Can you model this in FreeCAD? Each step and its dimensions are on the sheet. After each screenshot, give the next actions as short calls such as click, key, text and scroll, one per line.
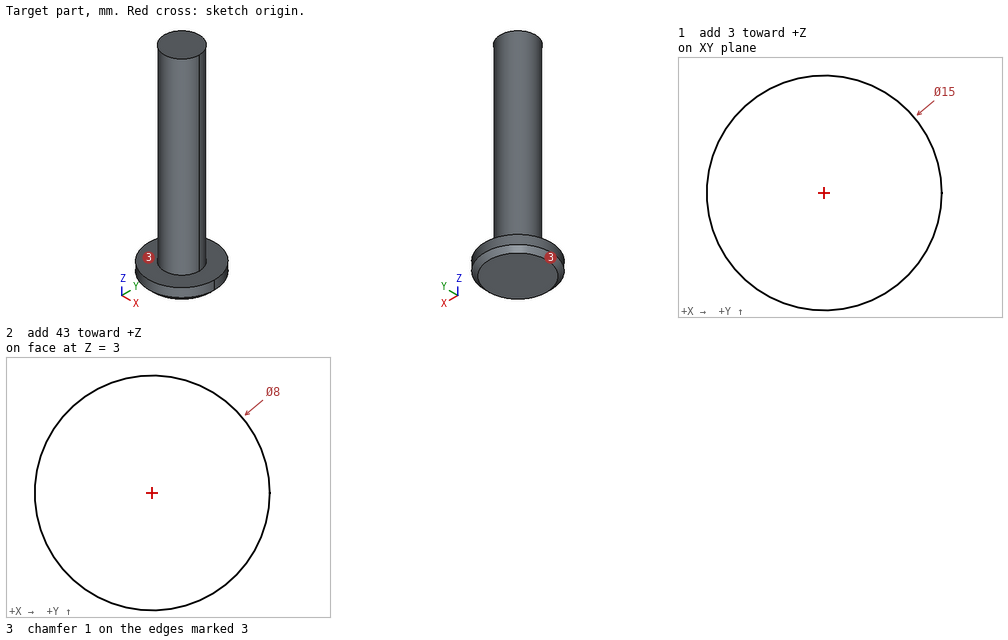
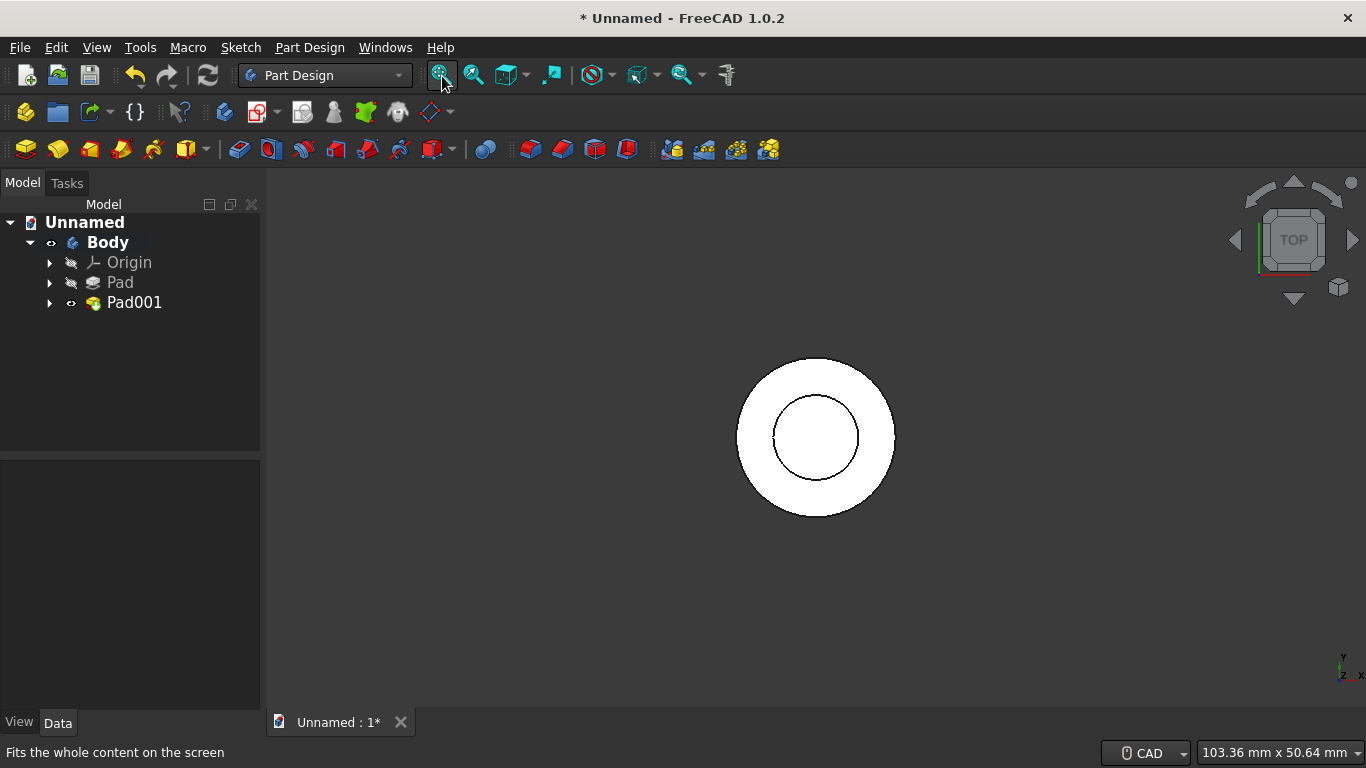
click(442, 76)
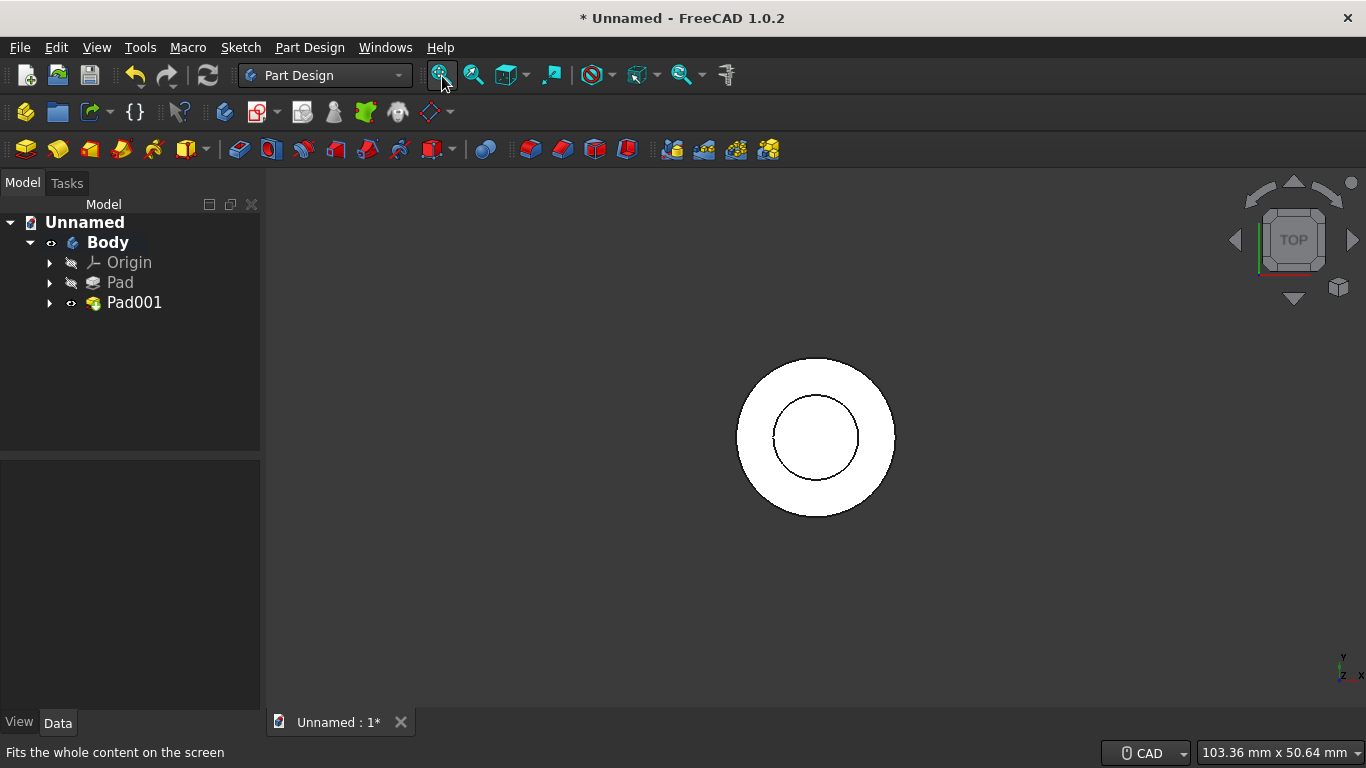
key(1)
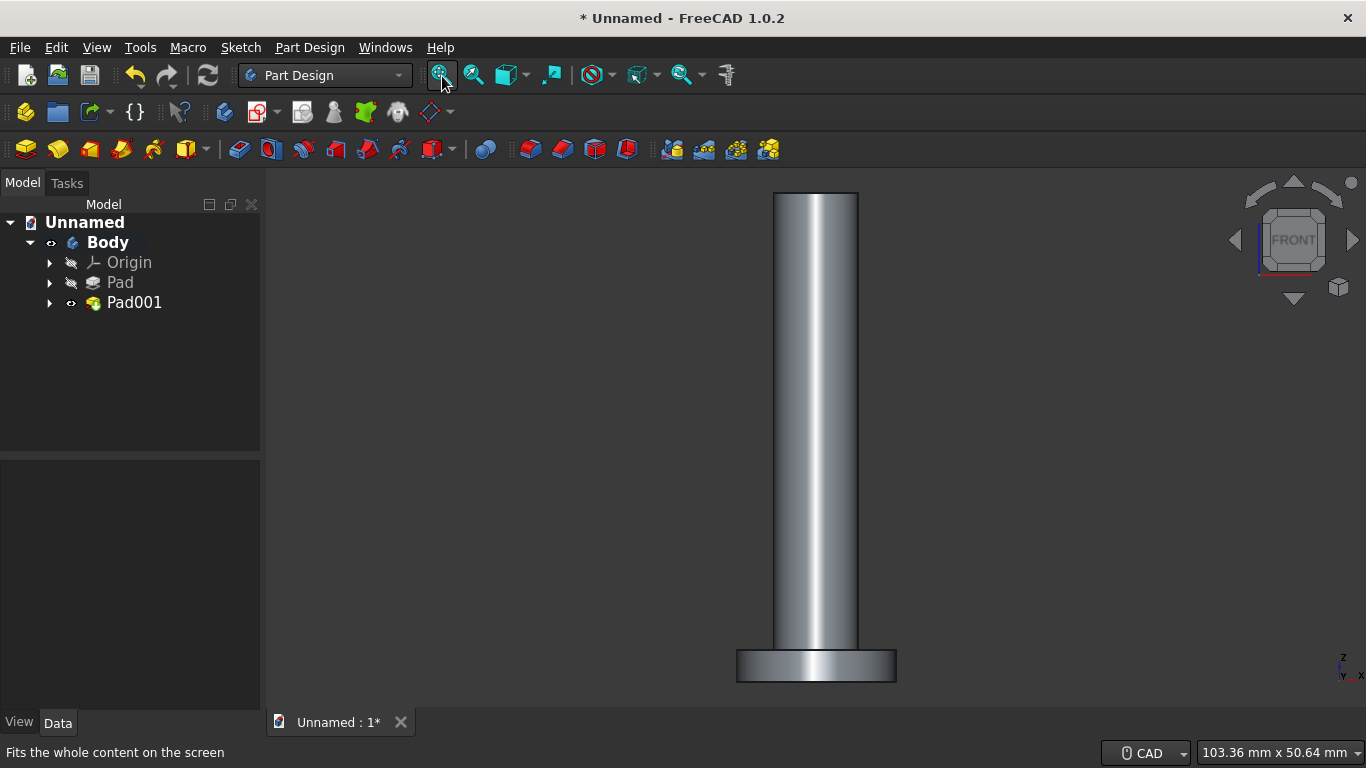
key(3)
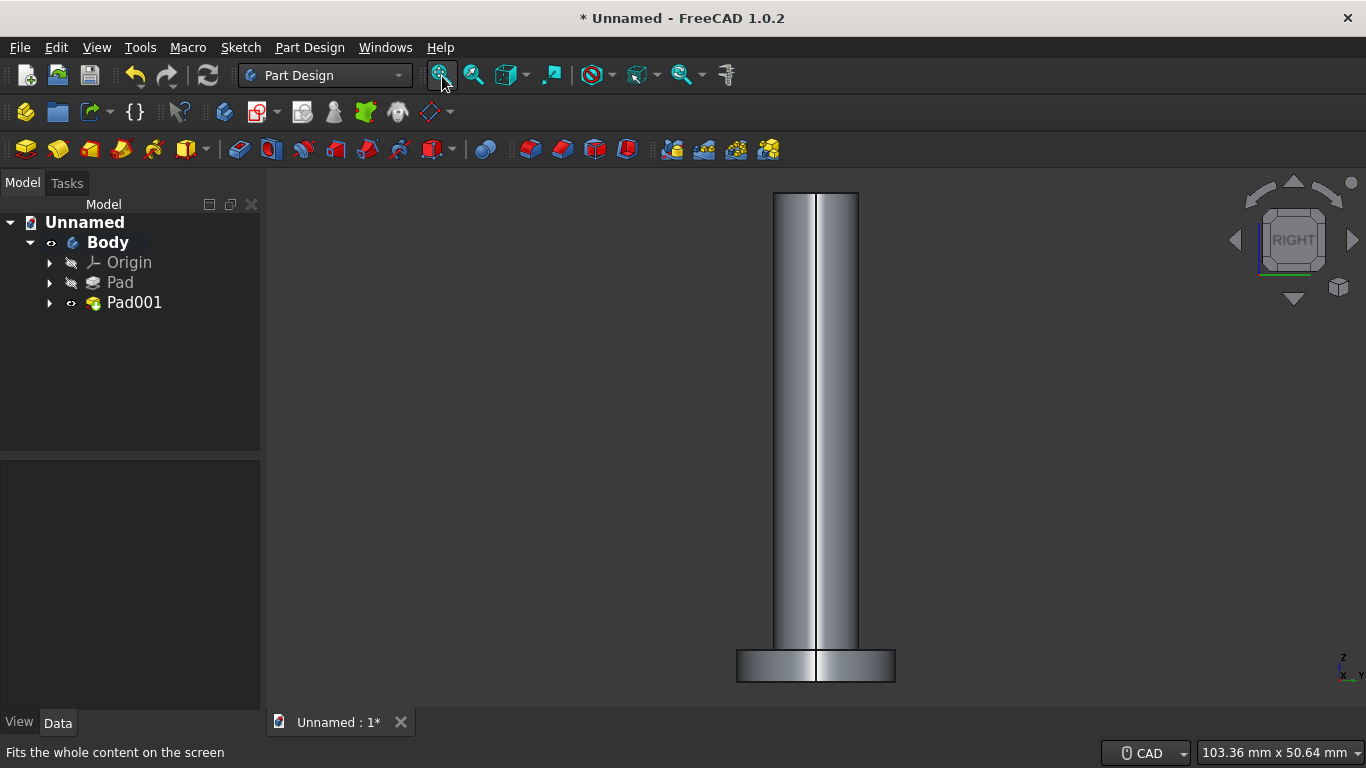
key(5)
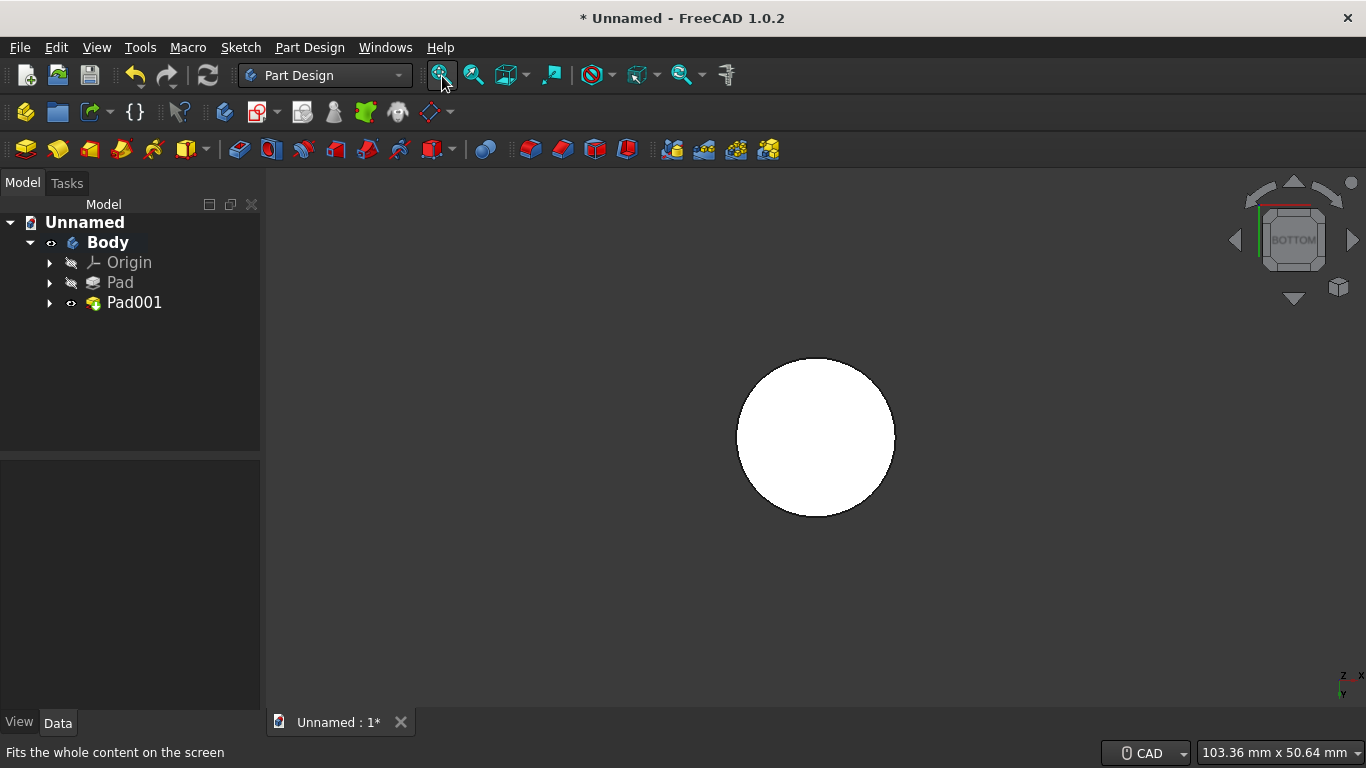
click(442, 76)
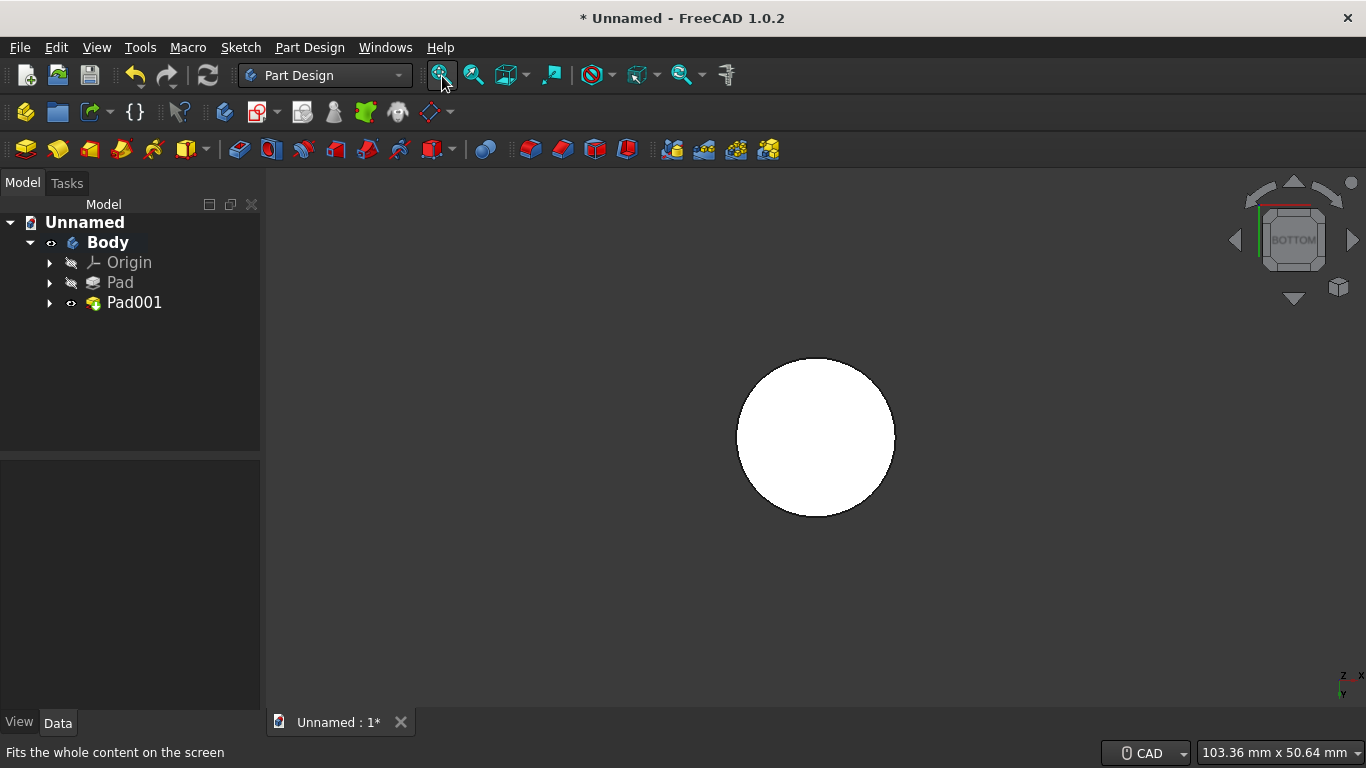
click(736, 436)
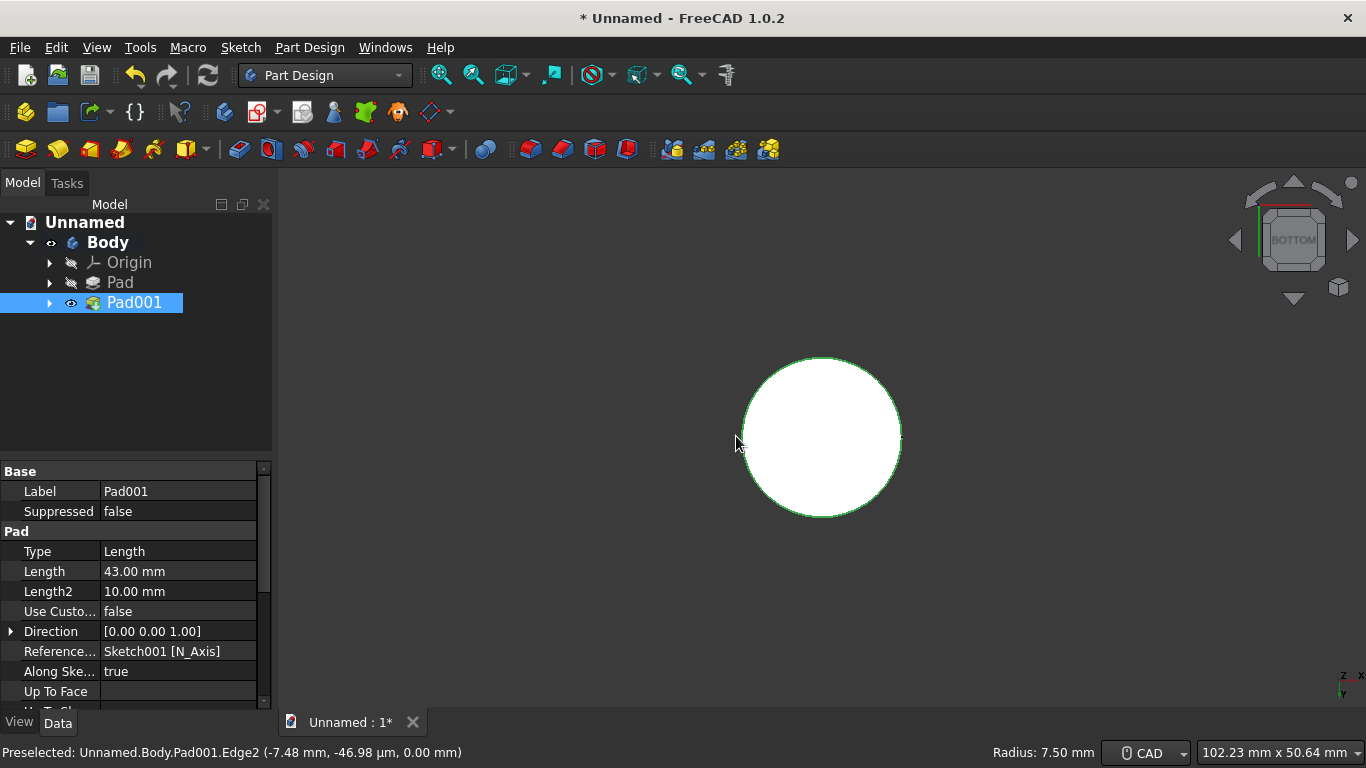
click(564, 150)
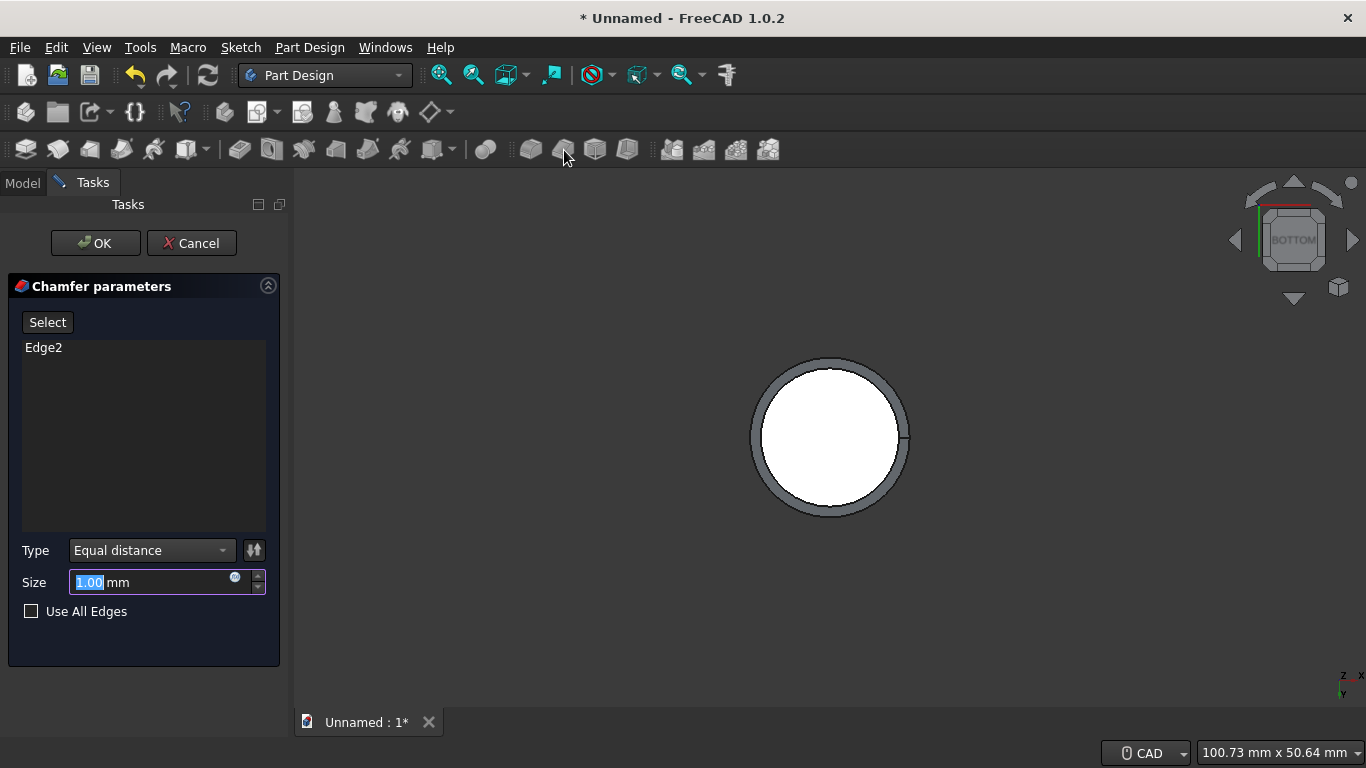
text(1)
key(Tab)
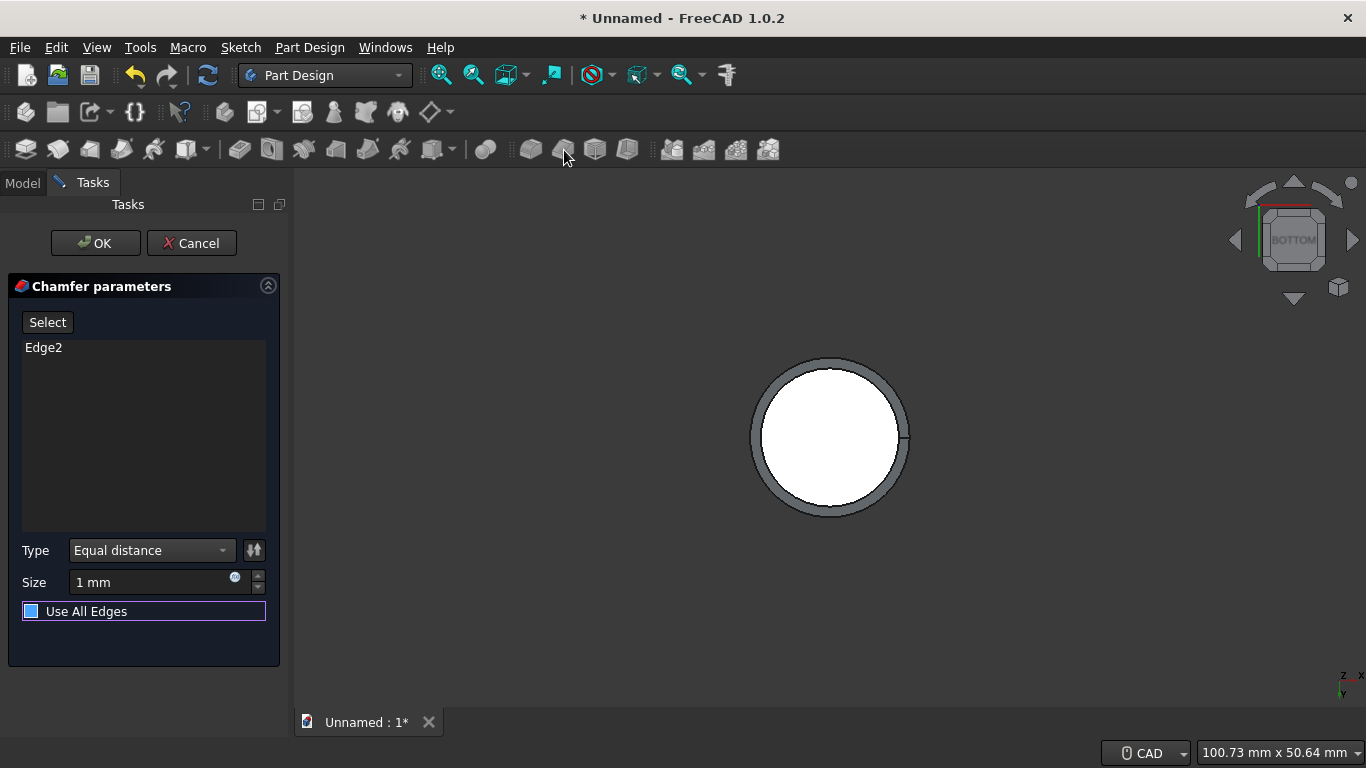
click(96, 243)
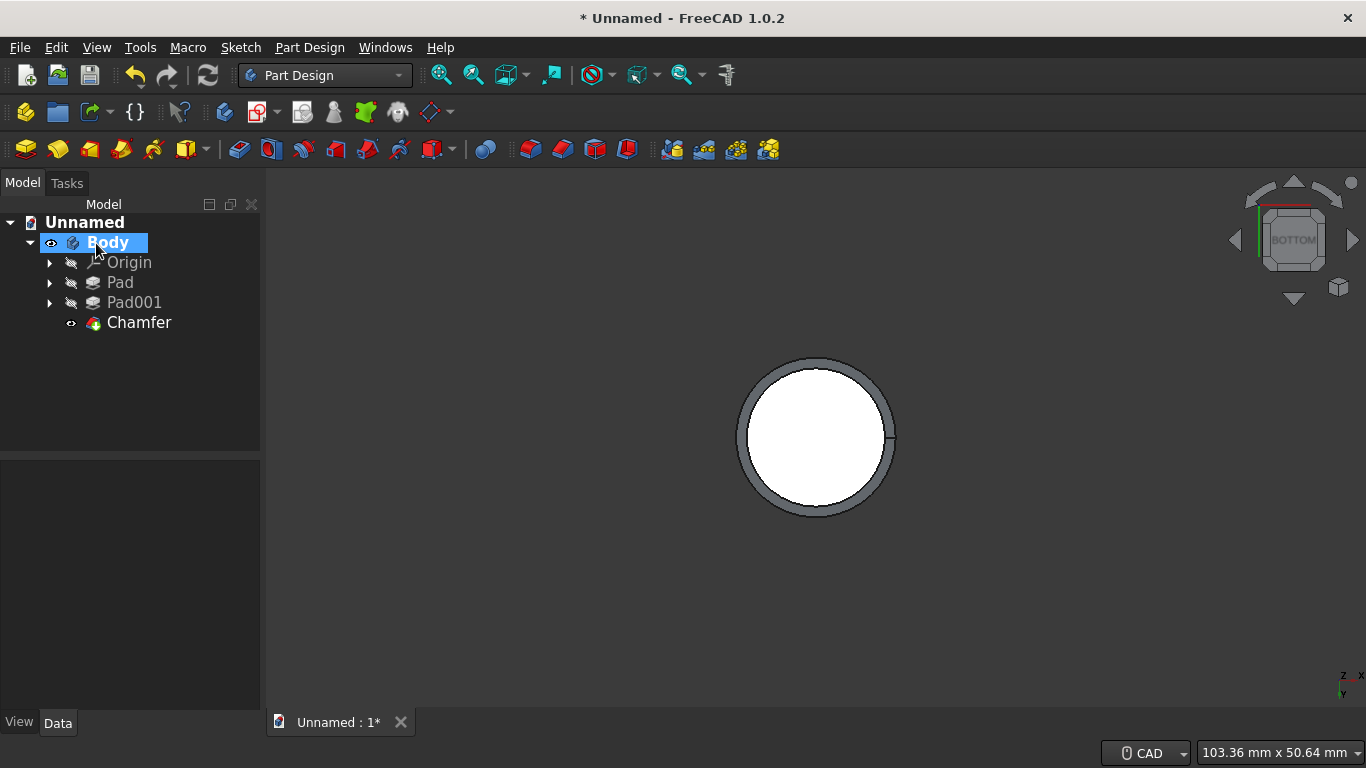
key(0)